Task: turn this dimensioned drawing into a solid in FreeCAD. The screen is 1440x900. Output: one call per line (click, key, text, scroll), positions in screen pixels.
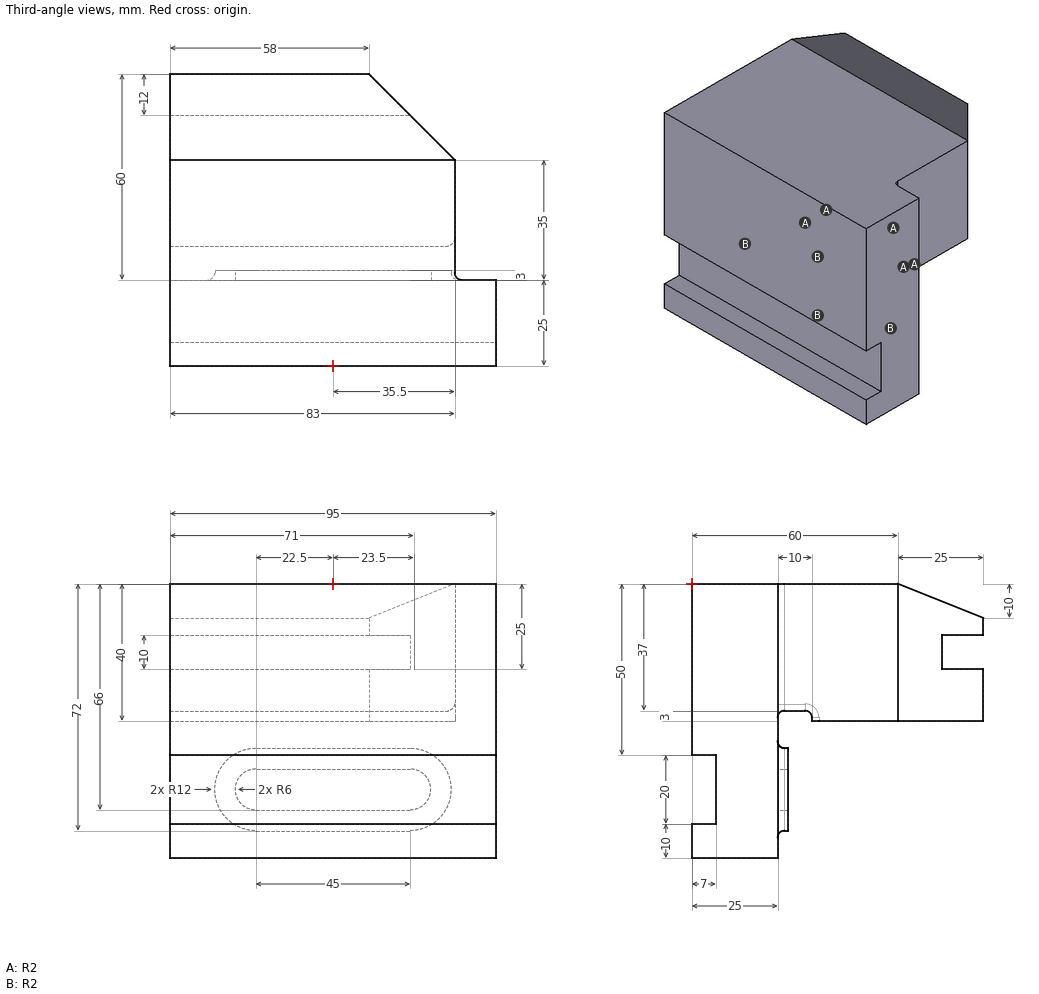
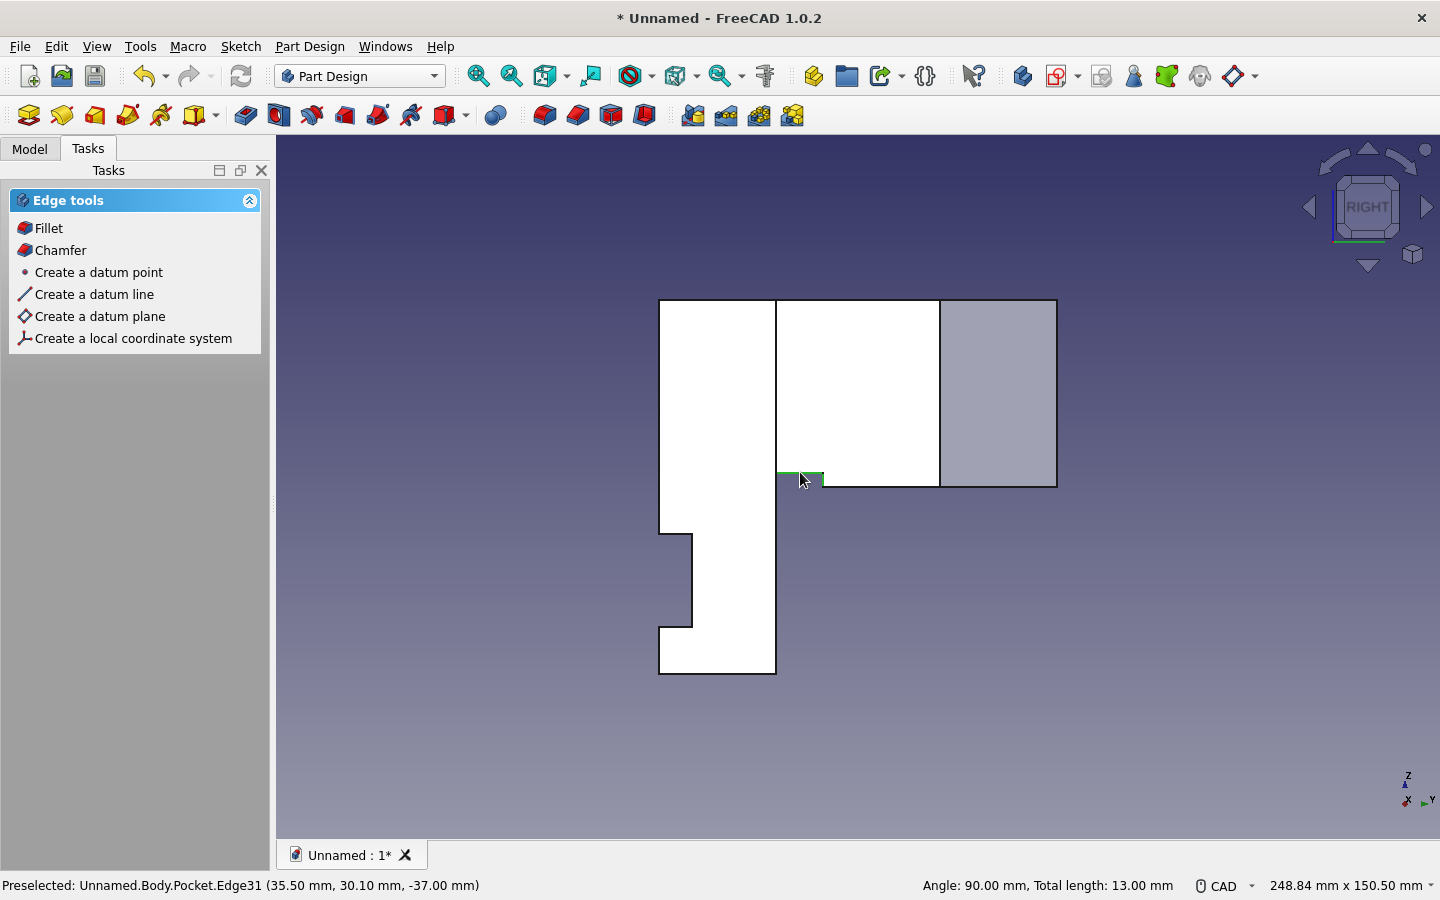
key(5)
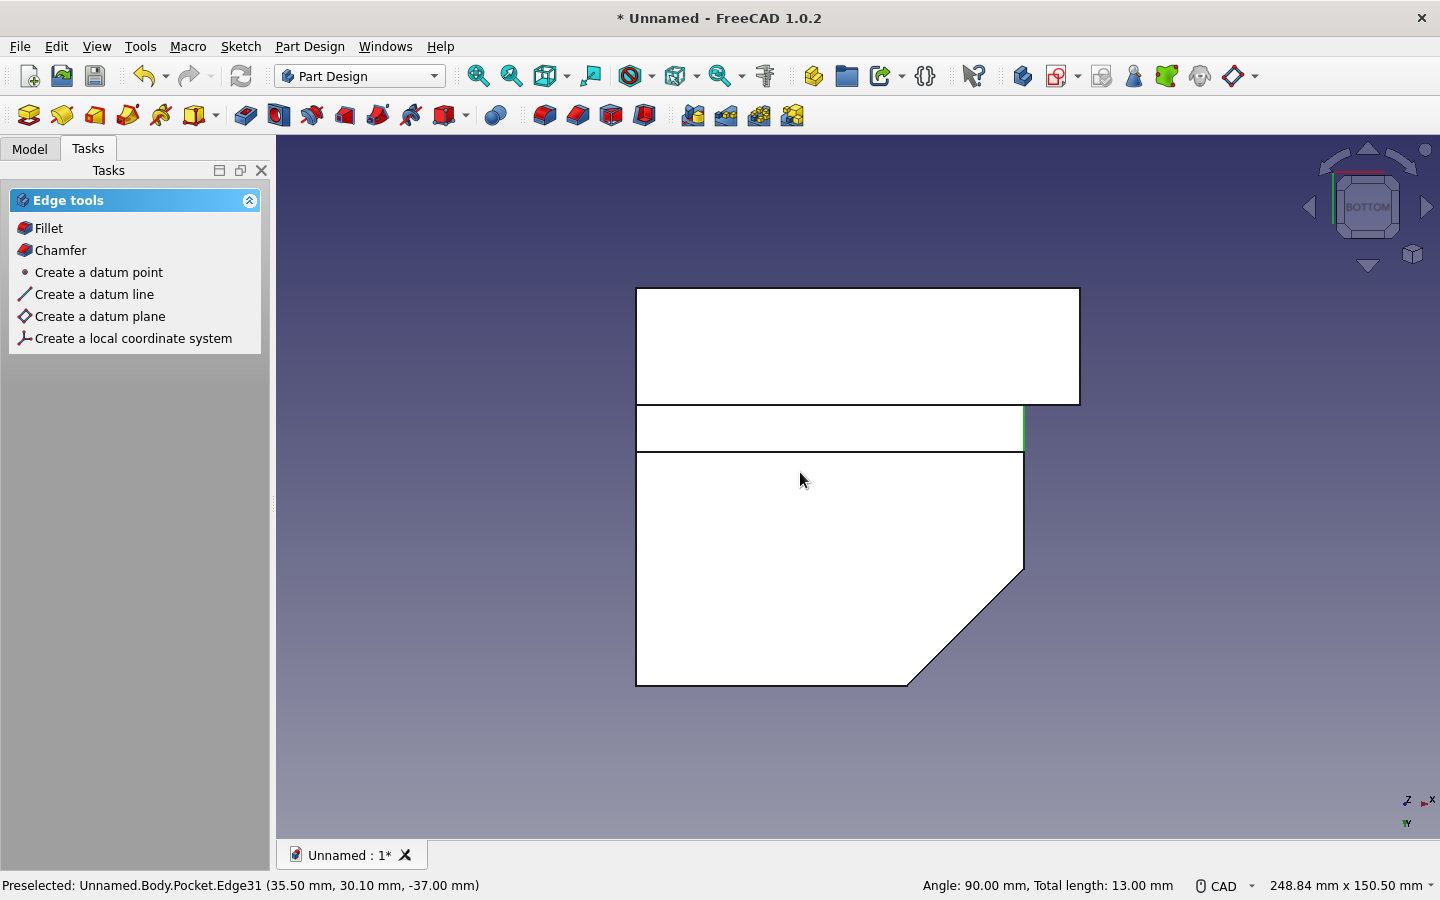
key(4)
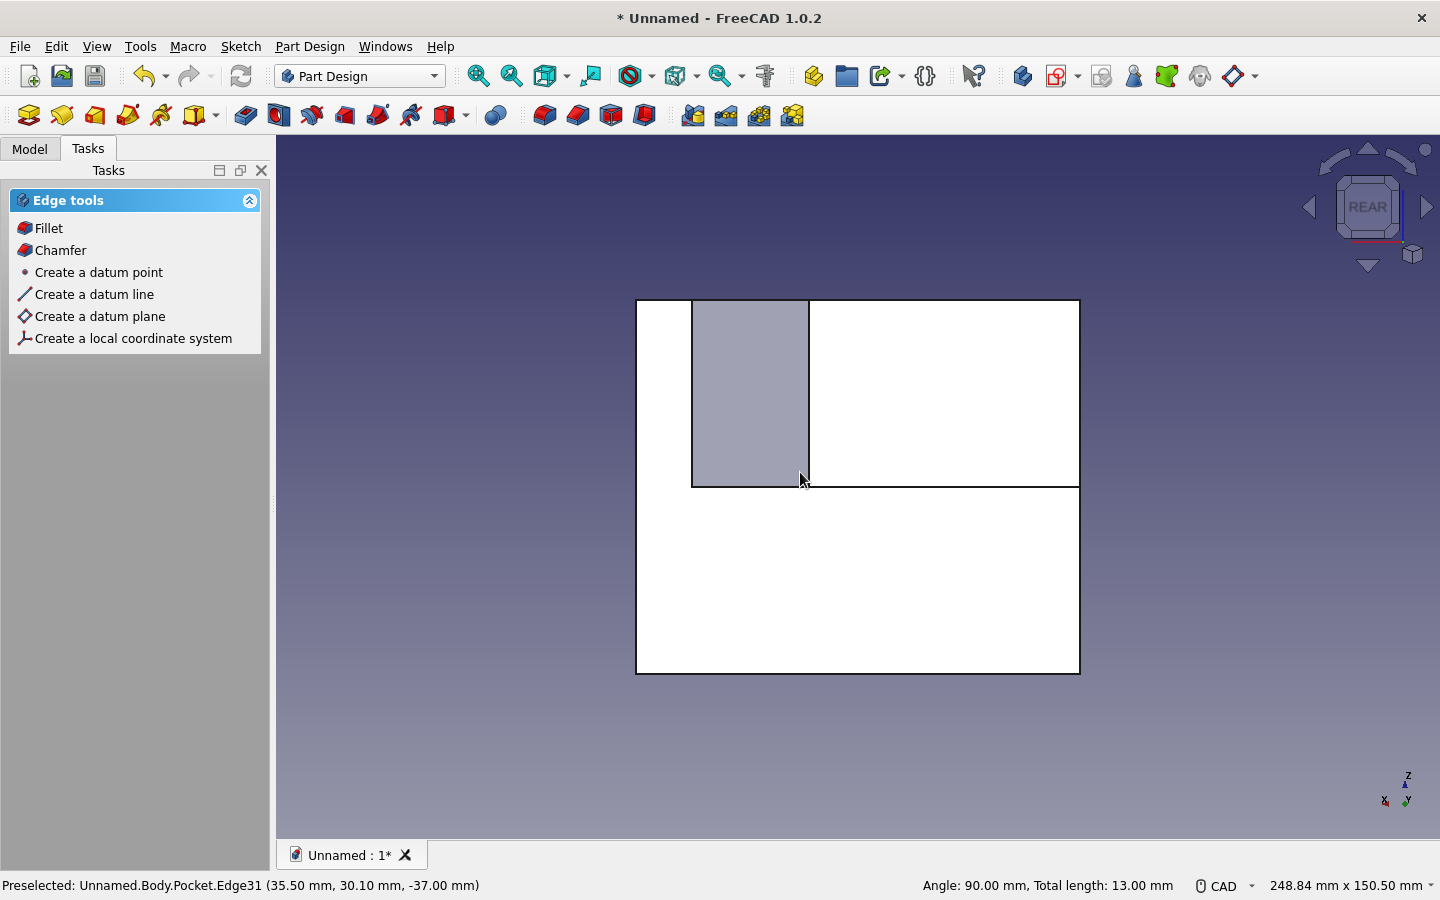
key(6)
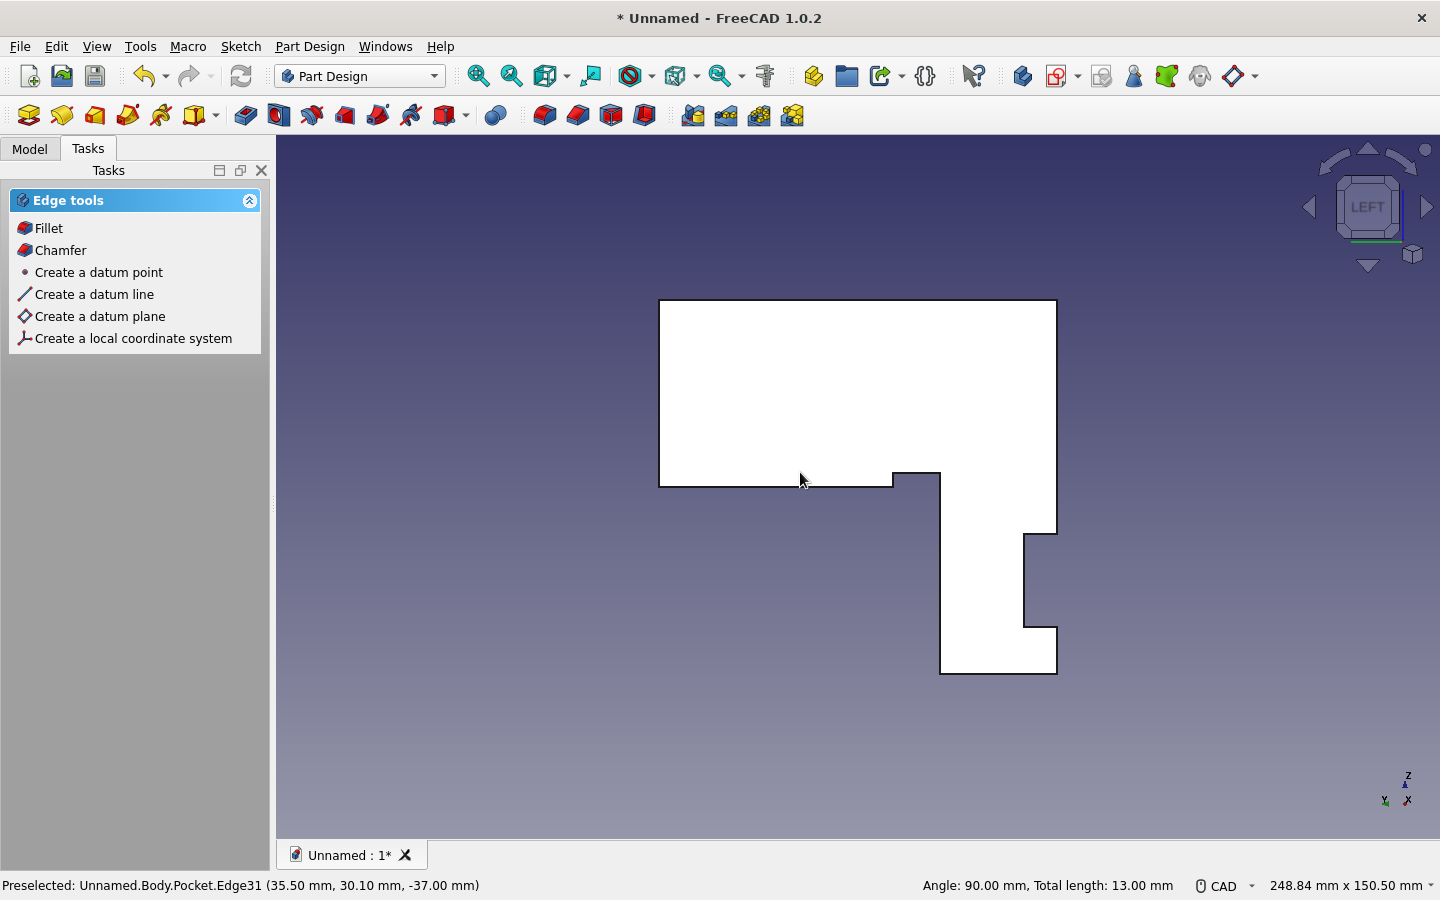
key(v)
key(3)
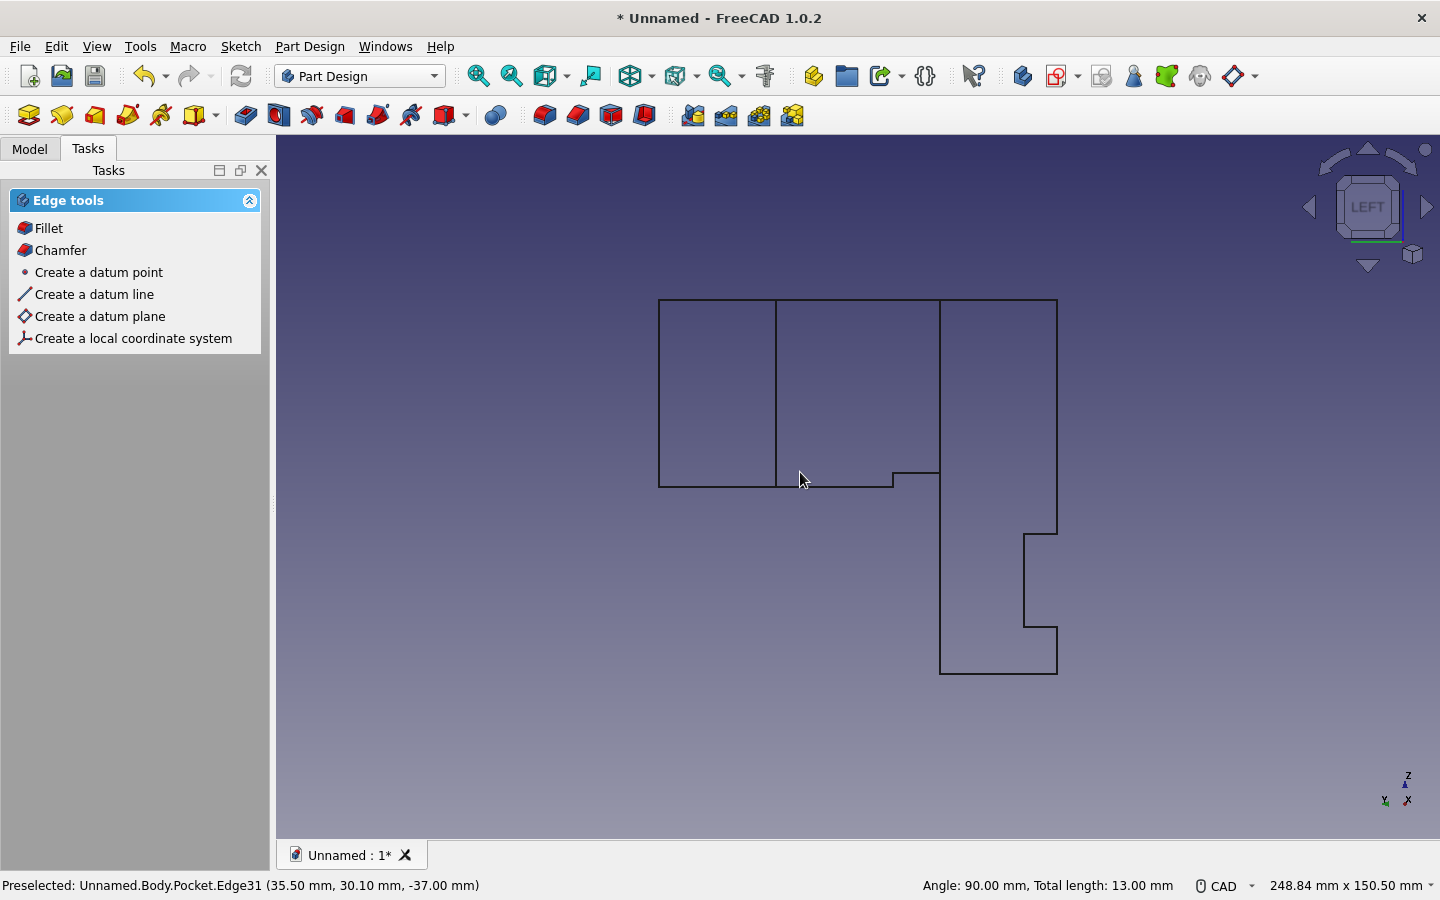
key(0)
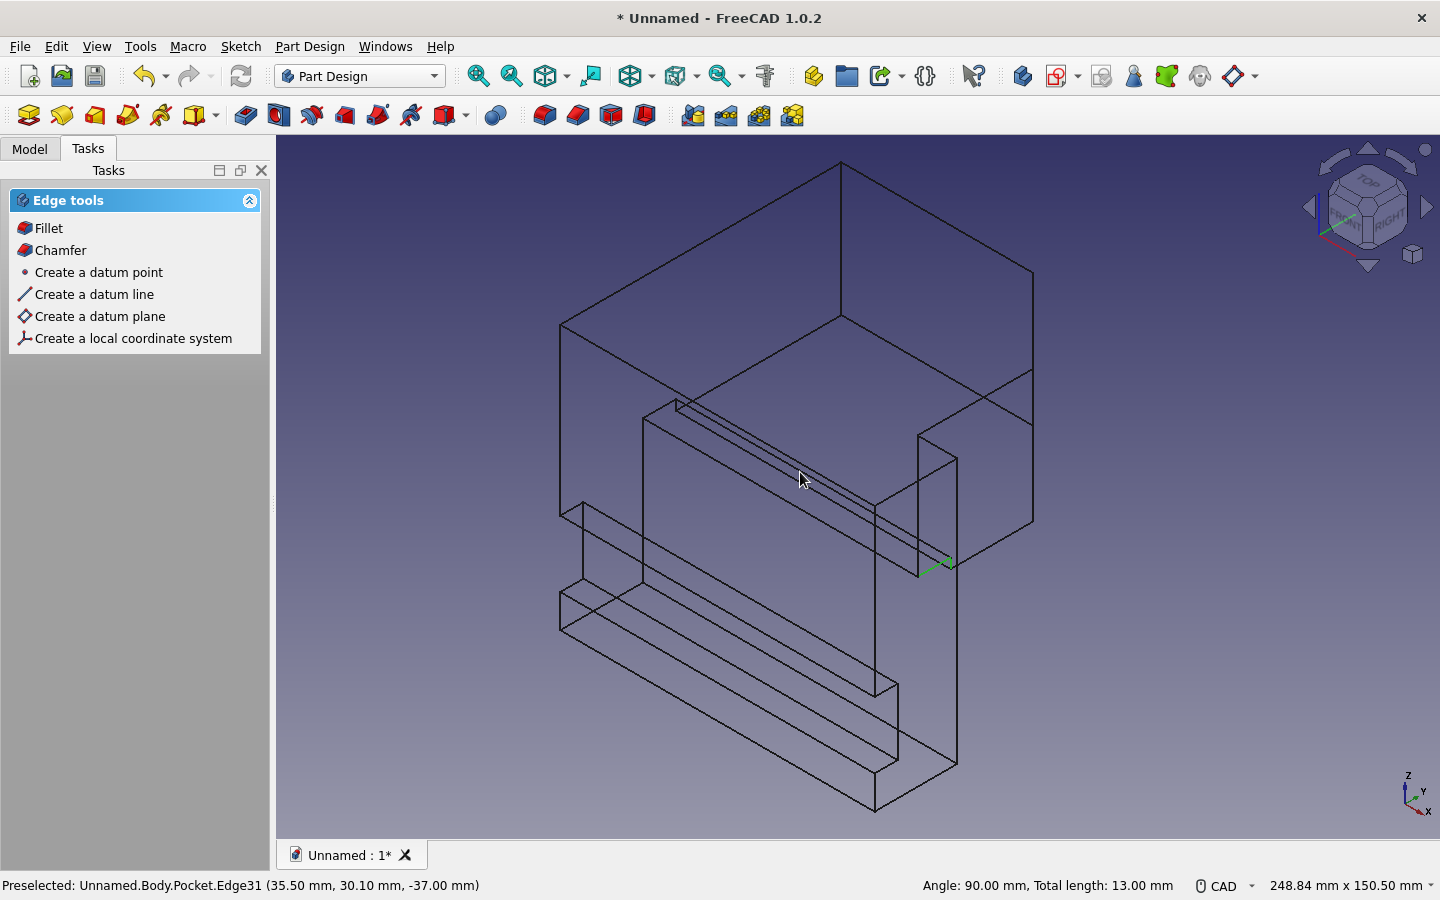
click(918, 505, ctrl)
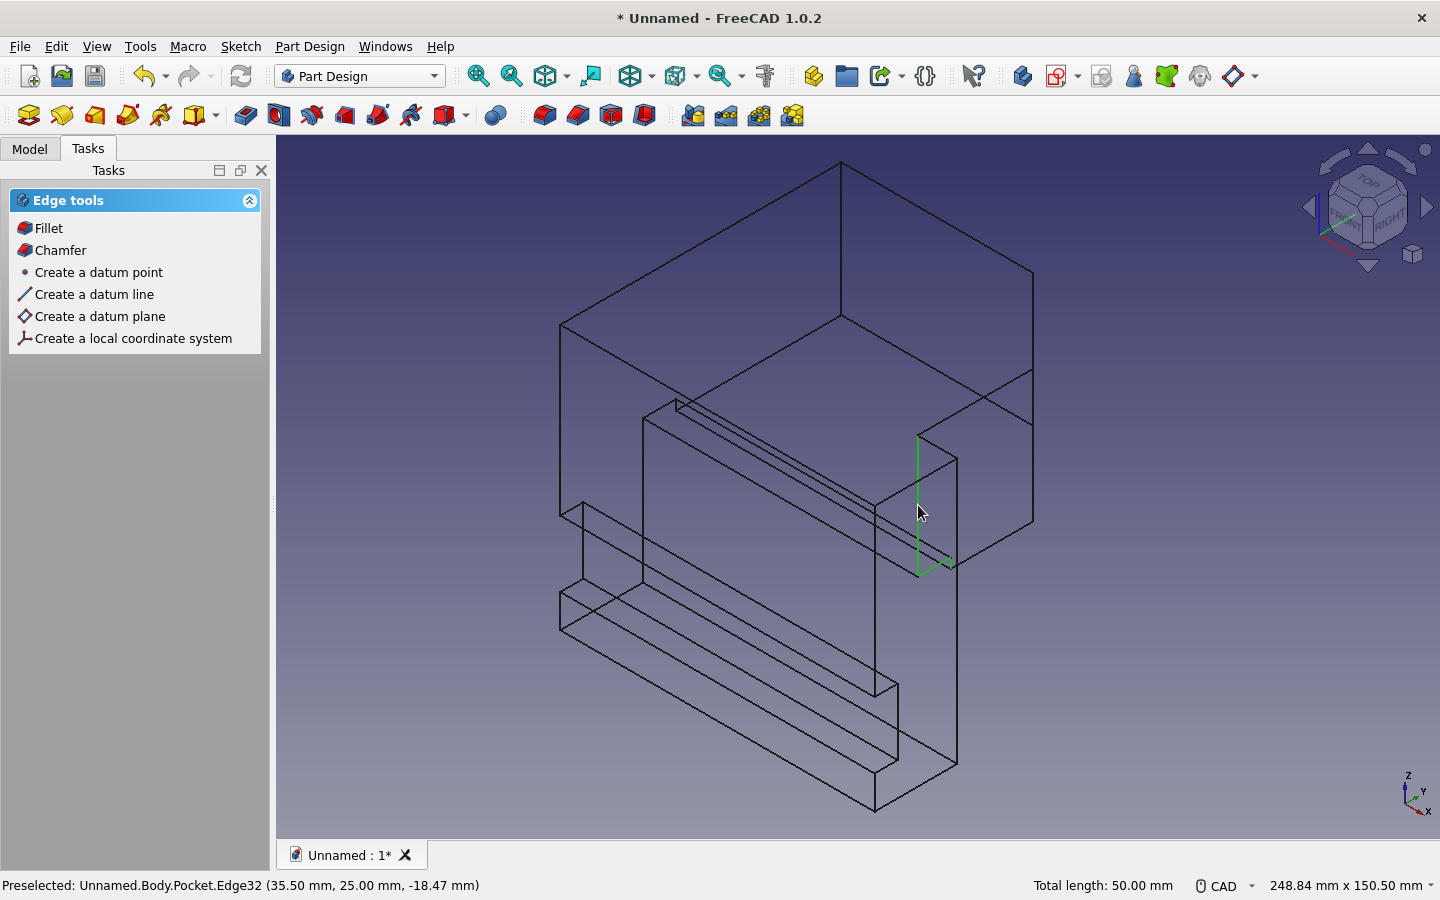
click(780, 497, ctrl)